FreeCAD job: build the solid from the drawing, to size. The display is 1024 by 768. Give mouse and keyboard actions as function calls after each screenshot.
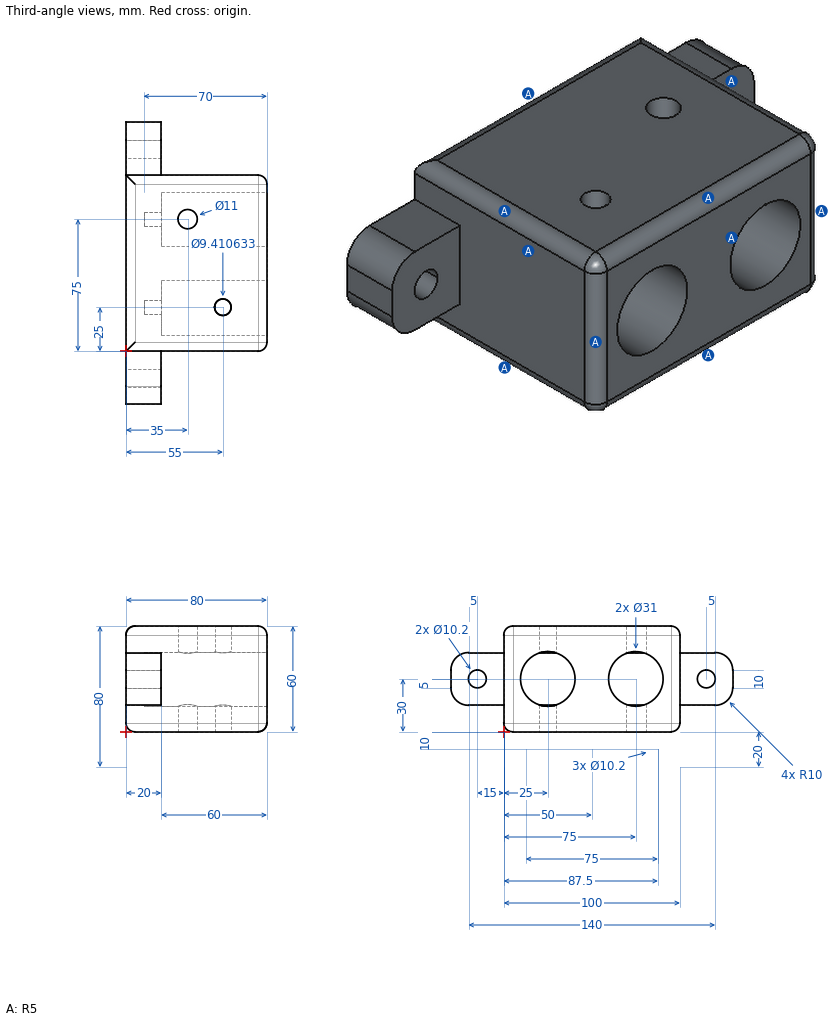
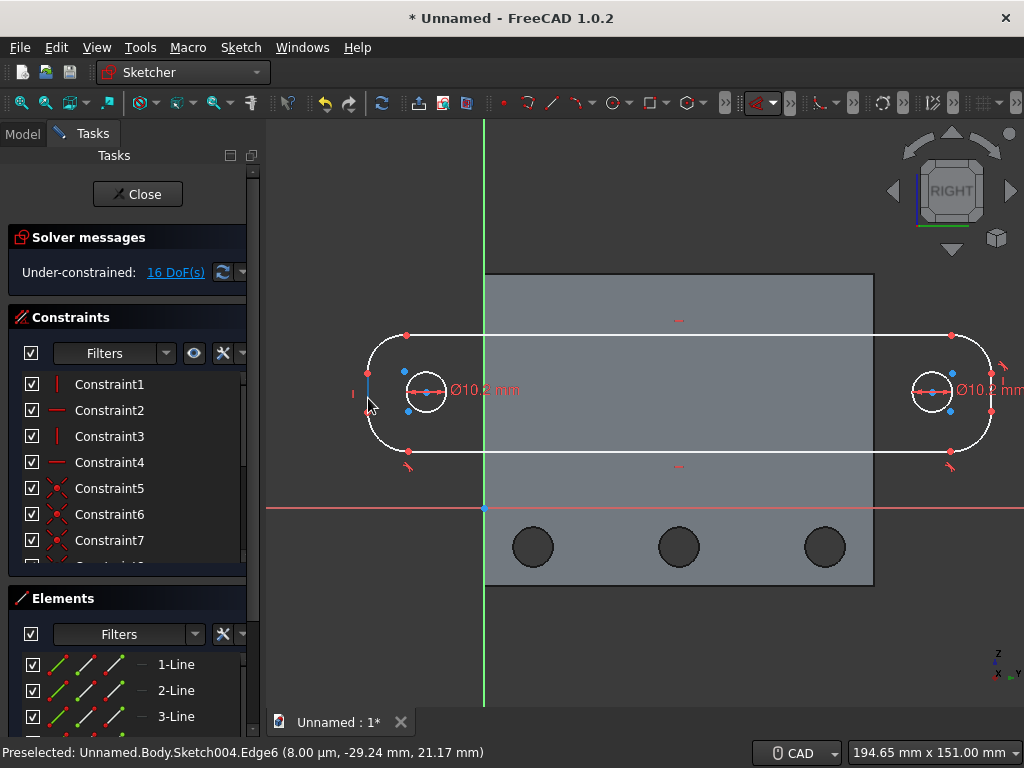
click(368, 397)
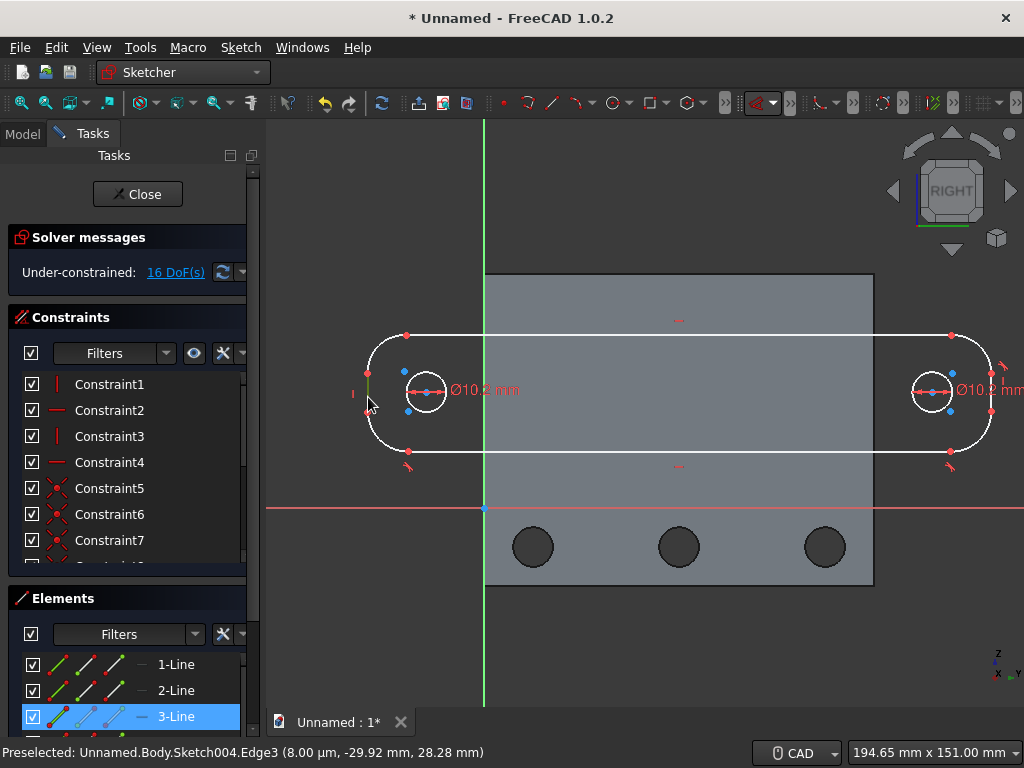
click(373, 430)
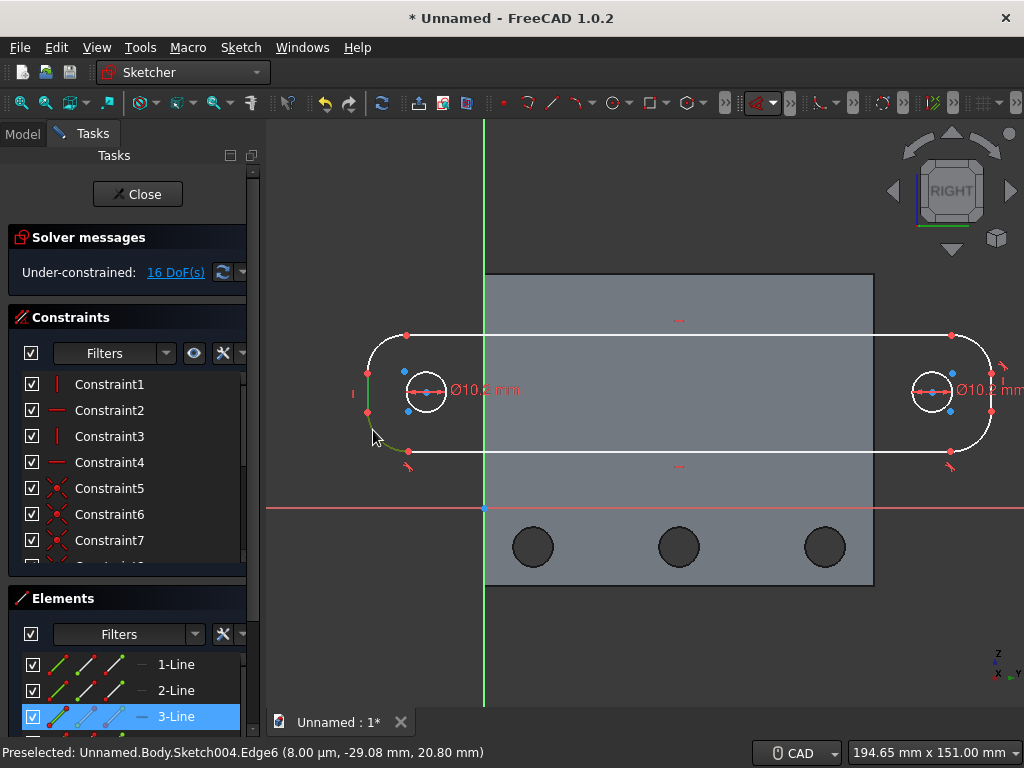
key(t)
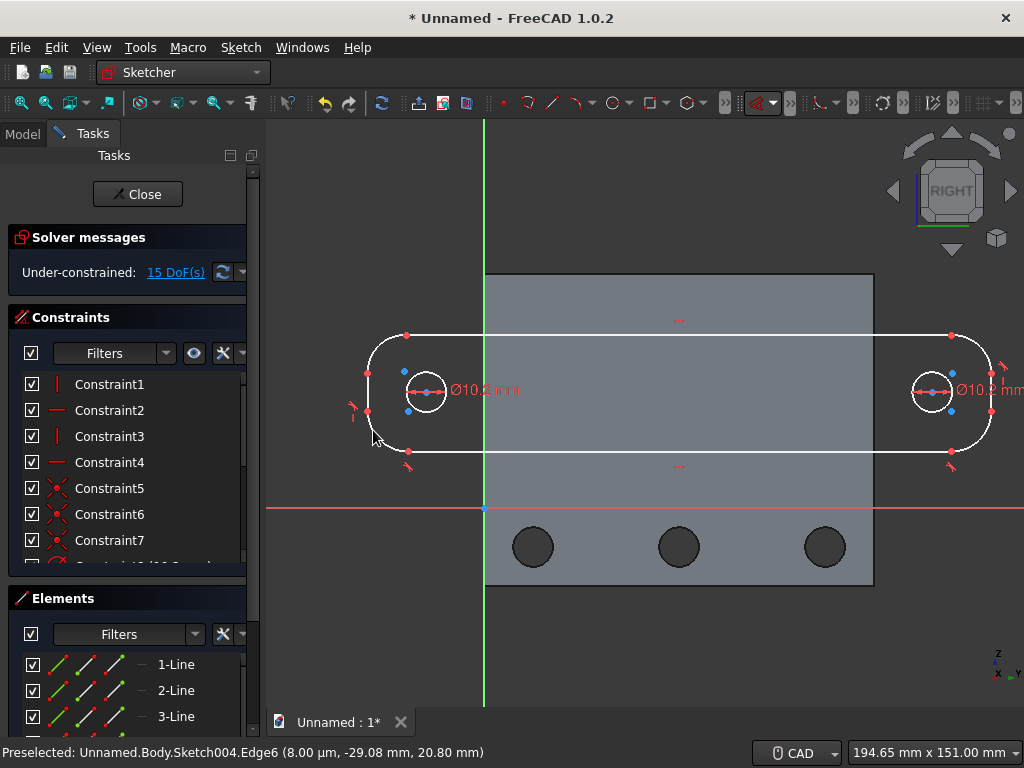
scroll(368, 400, up, 2)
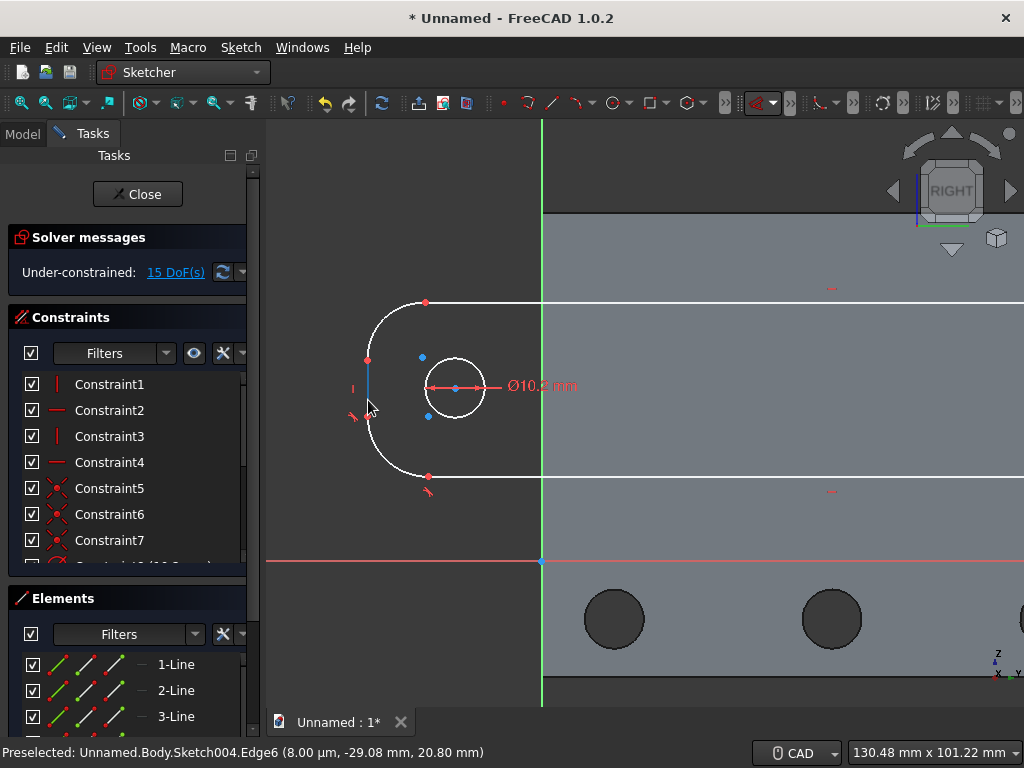
click(368, 400)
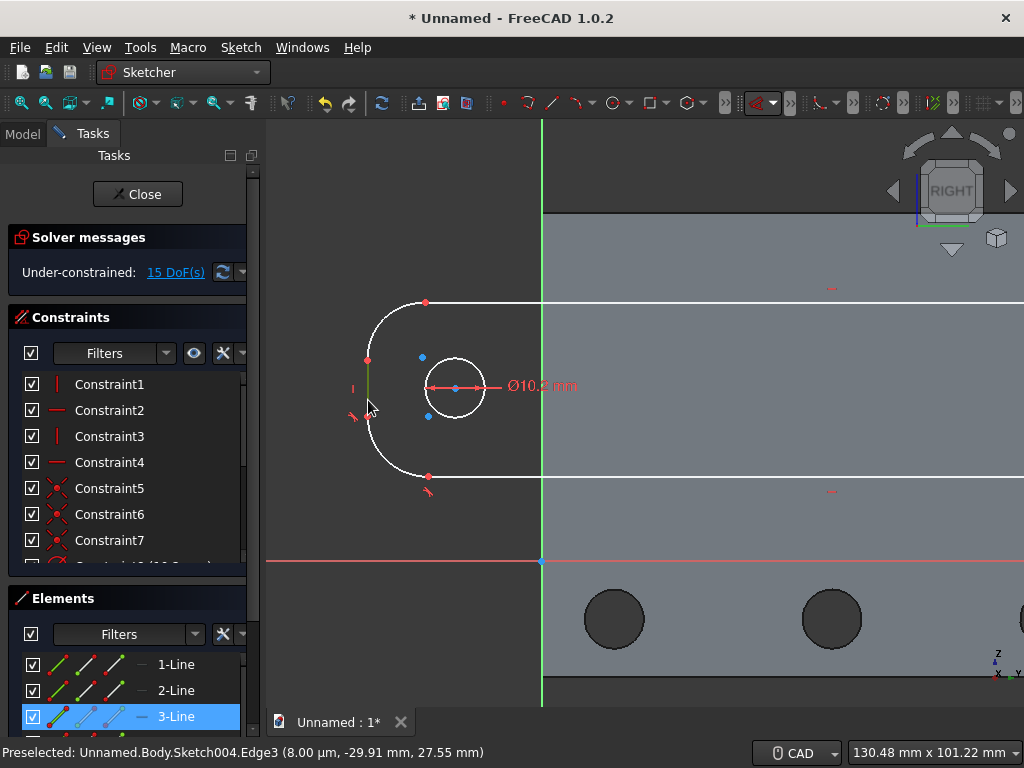
click(399, 308)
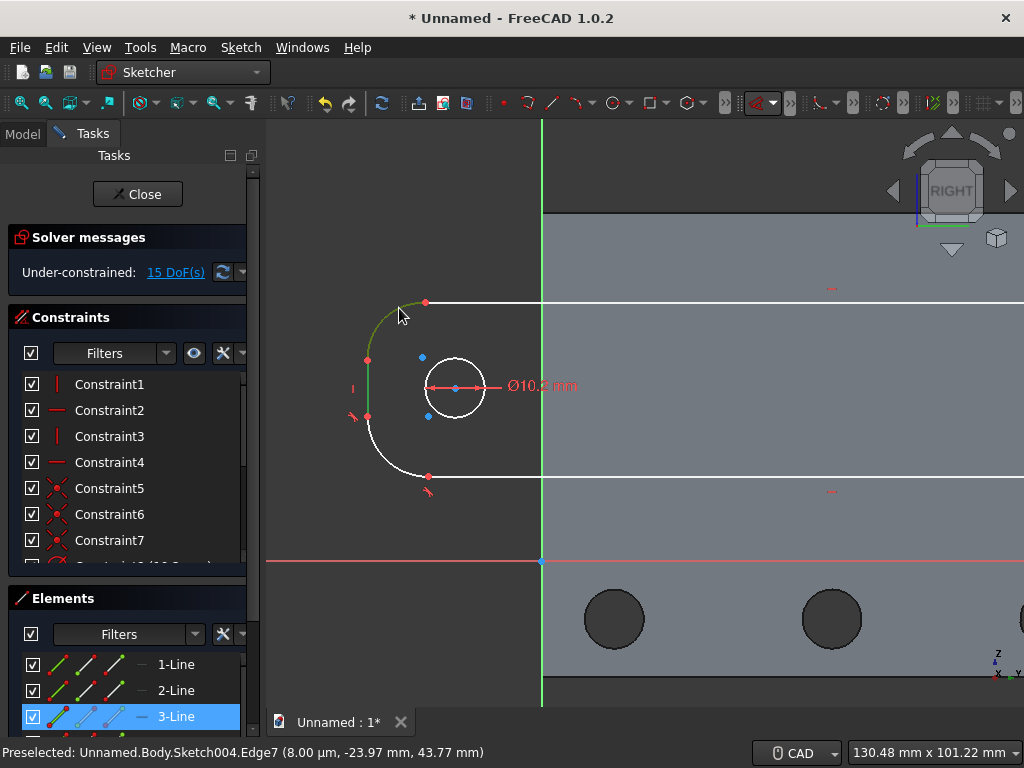
key(t)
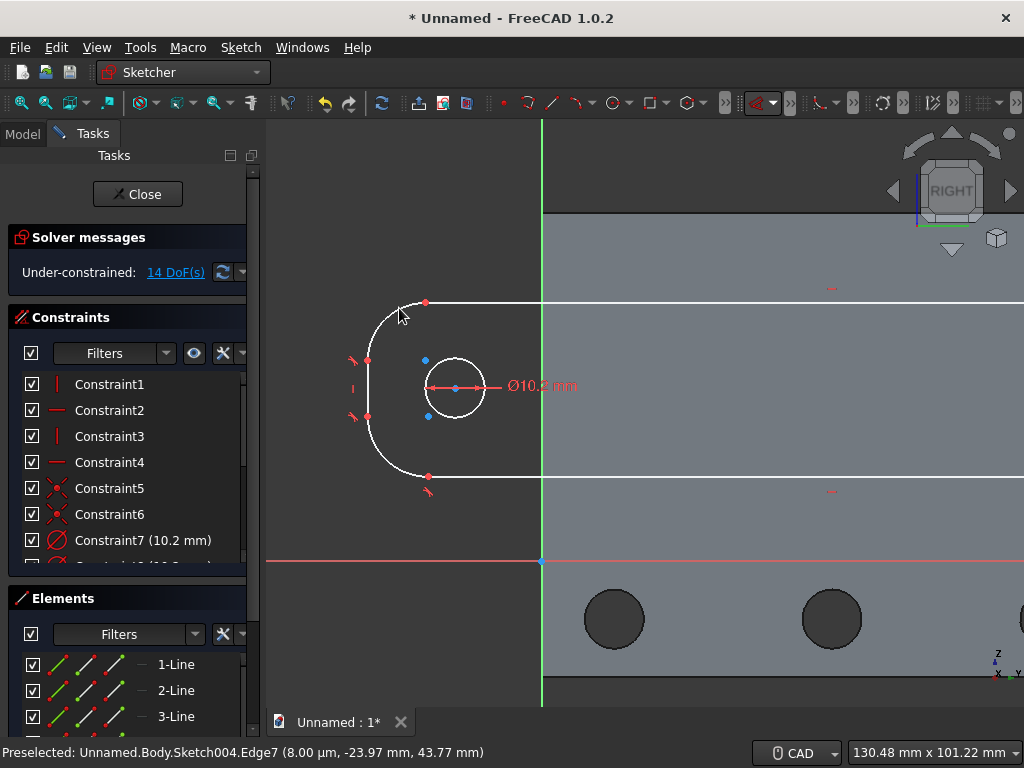
click(670, 303)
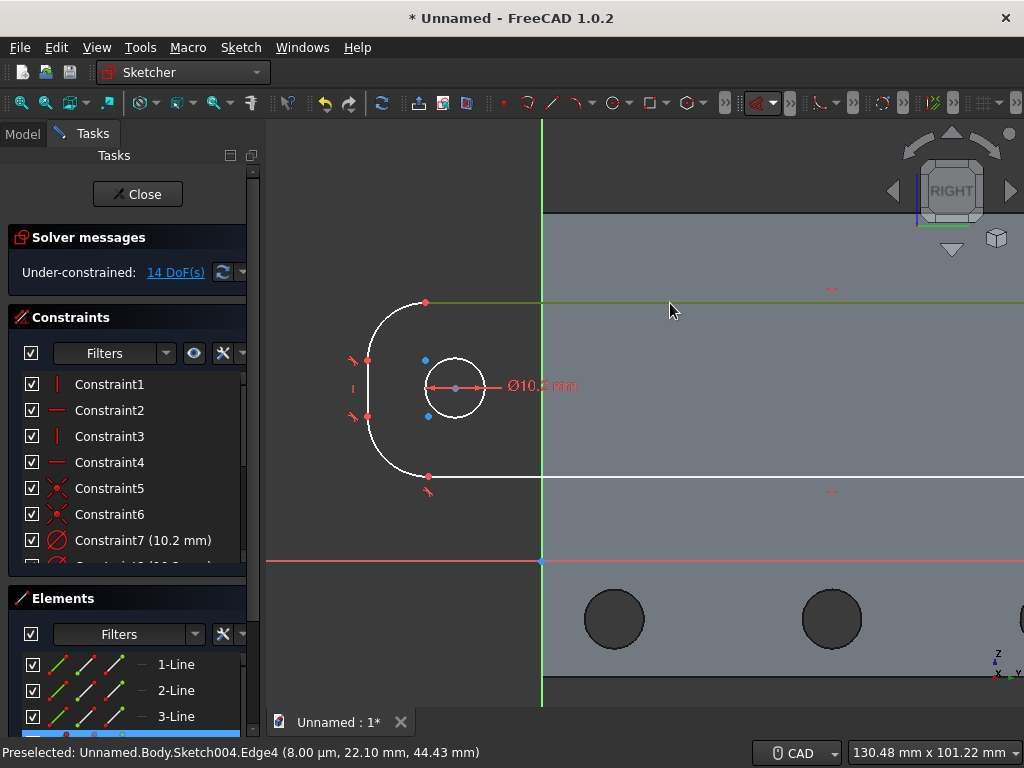
click(400, 309)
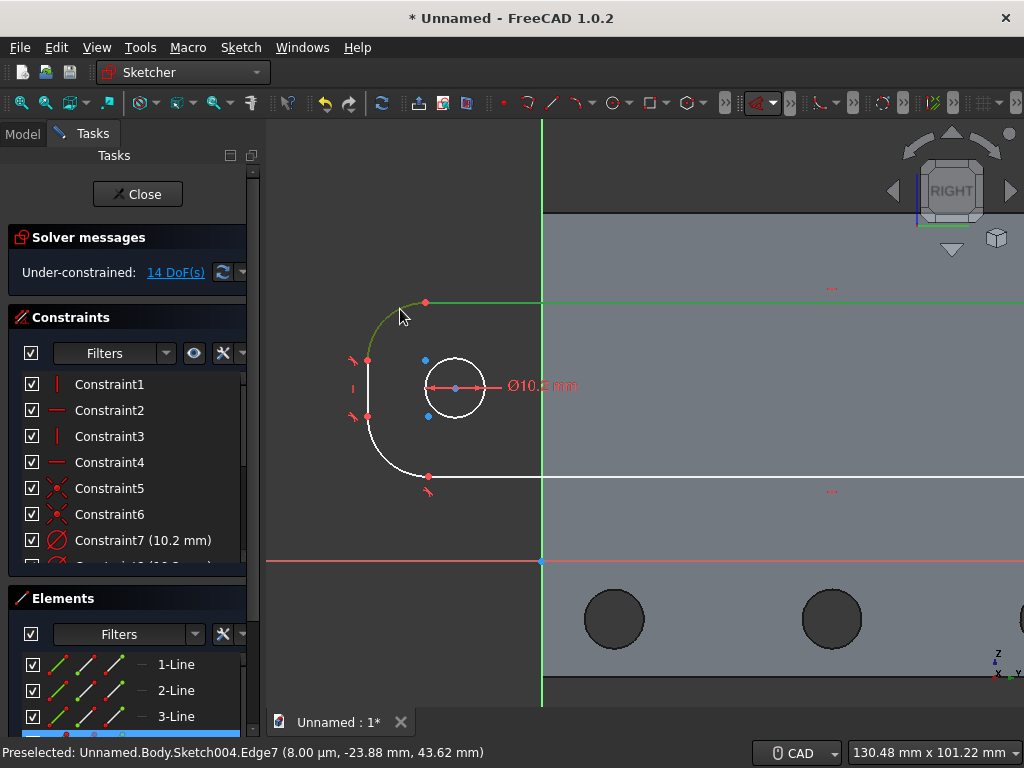
key(t)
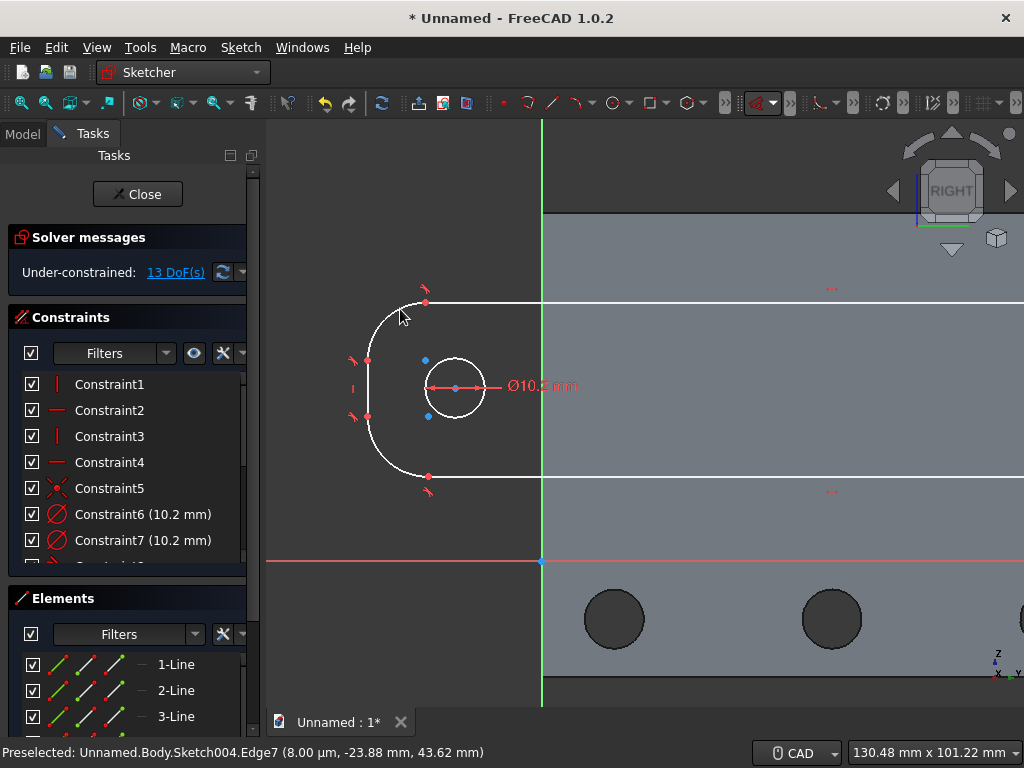
click(670, 303)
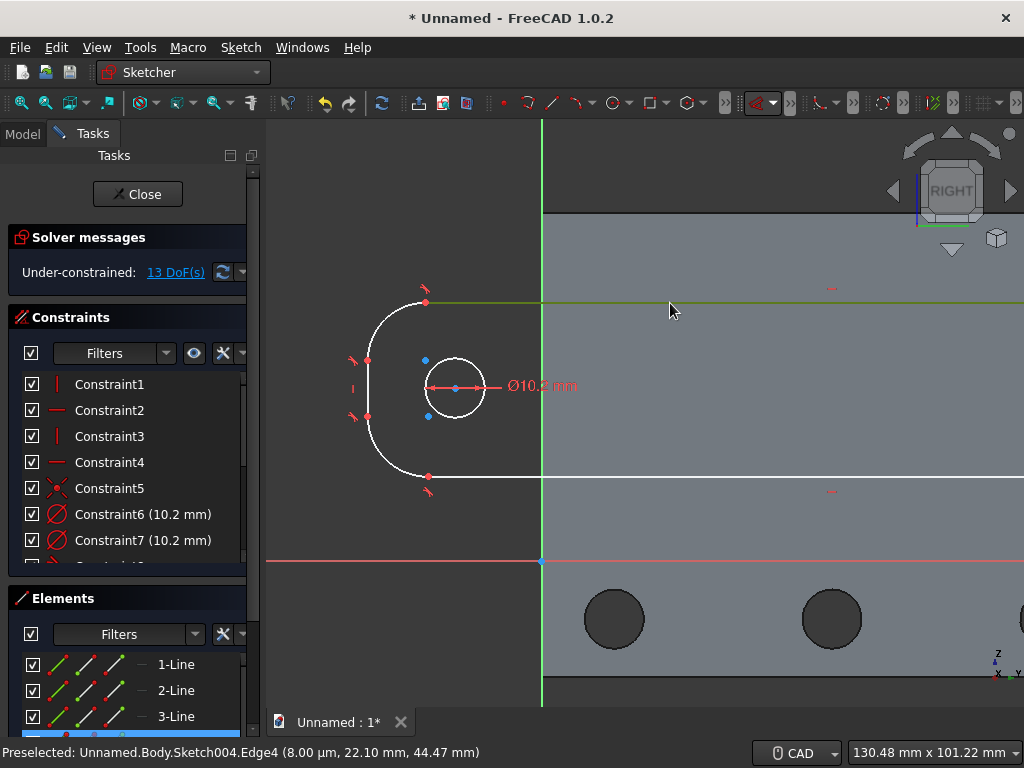
scroll(368, 399, down, 4)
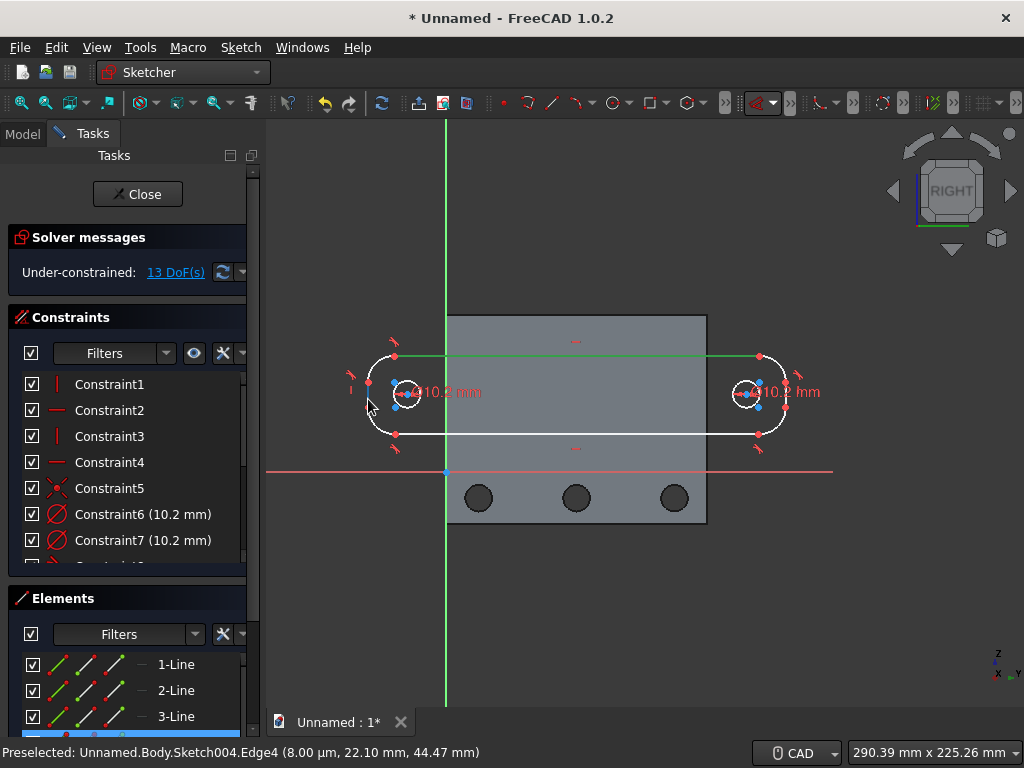
click(783, 370)